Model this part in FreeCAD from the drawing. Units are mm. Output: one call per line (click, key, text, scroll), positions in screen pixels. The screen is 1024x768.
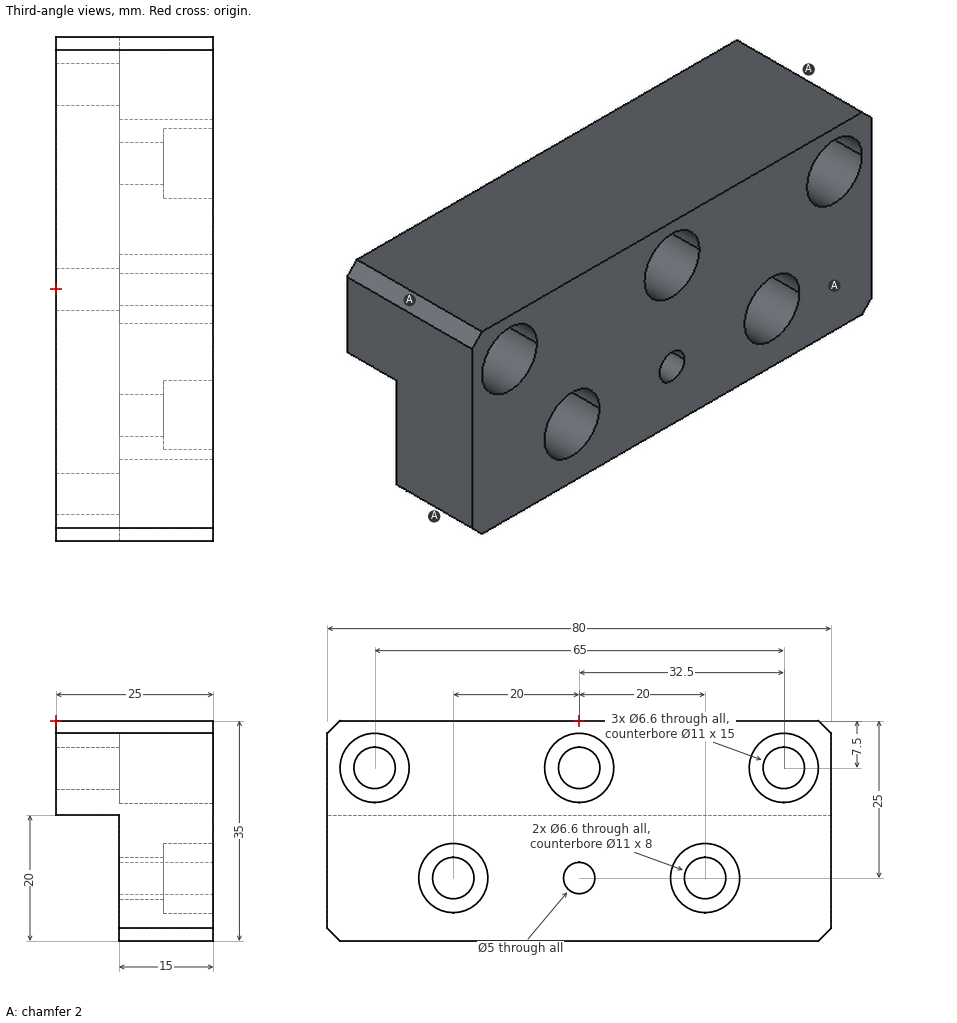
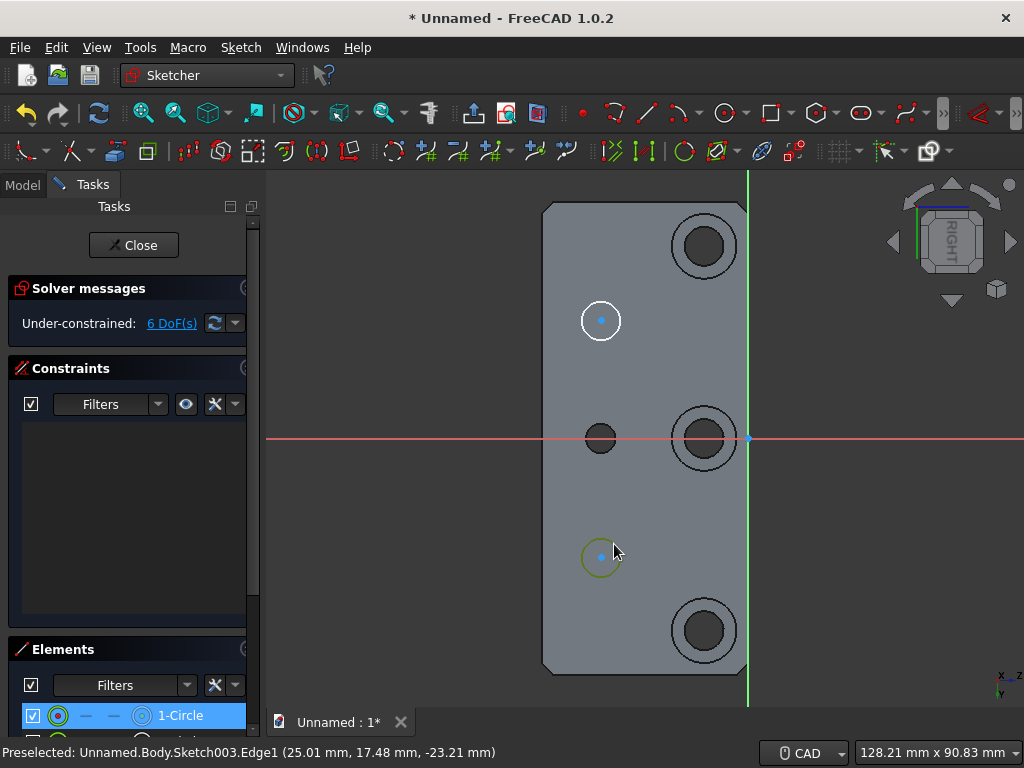
click(614, 307)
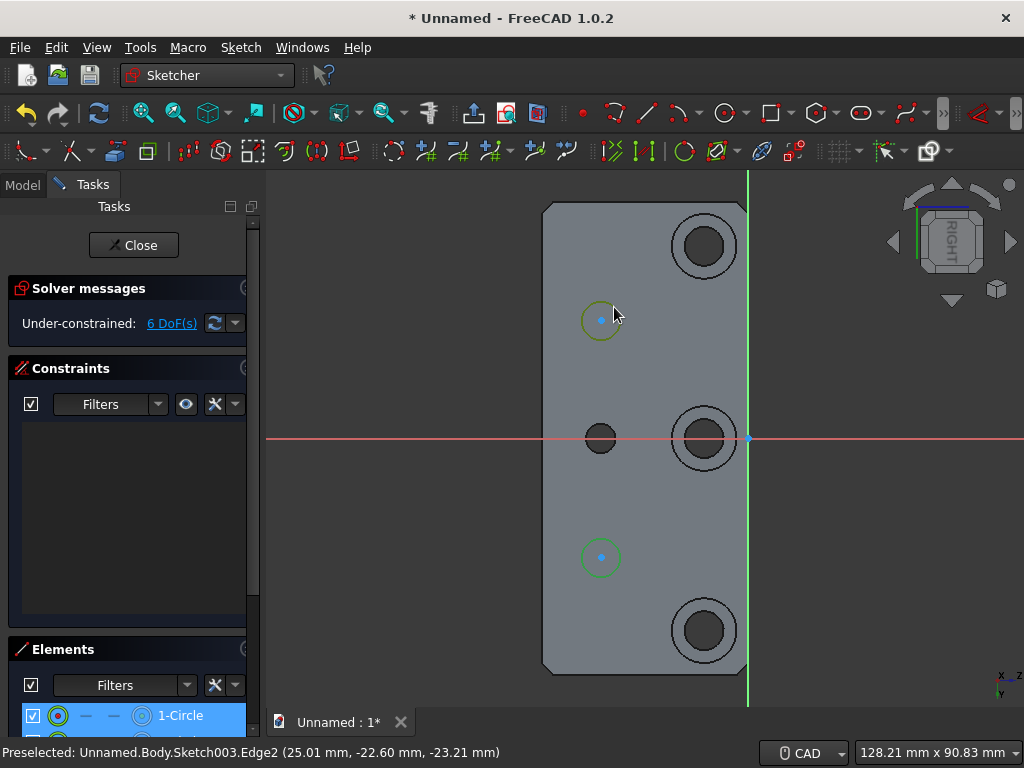
key(e)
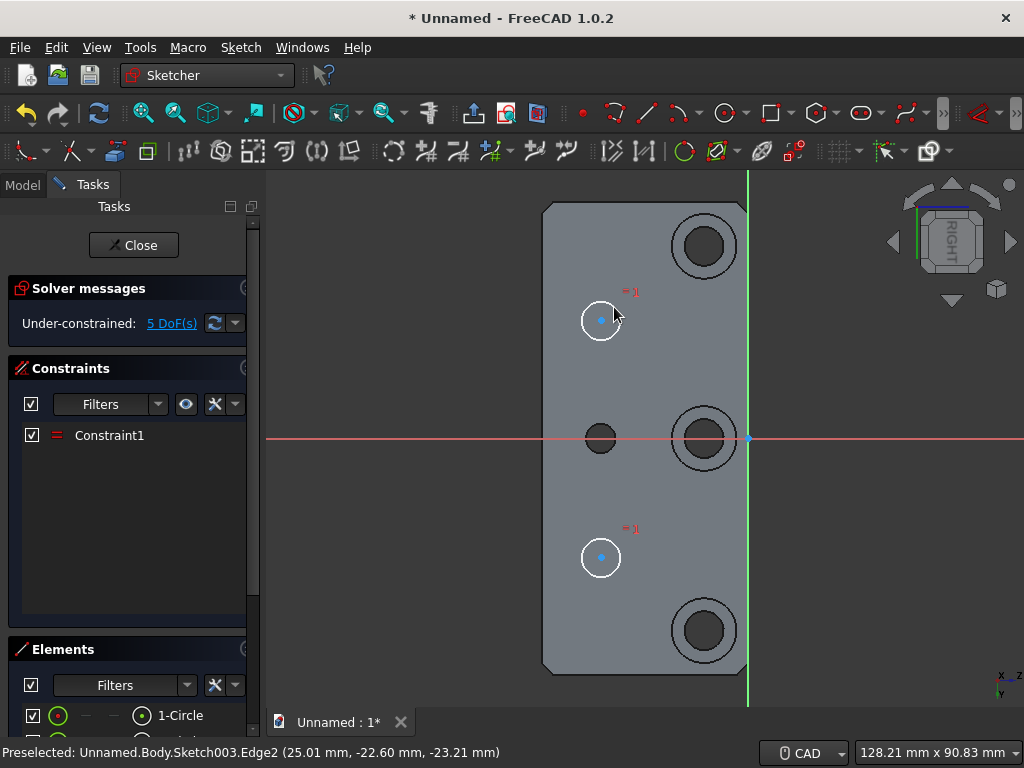
click(601, 558)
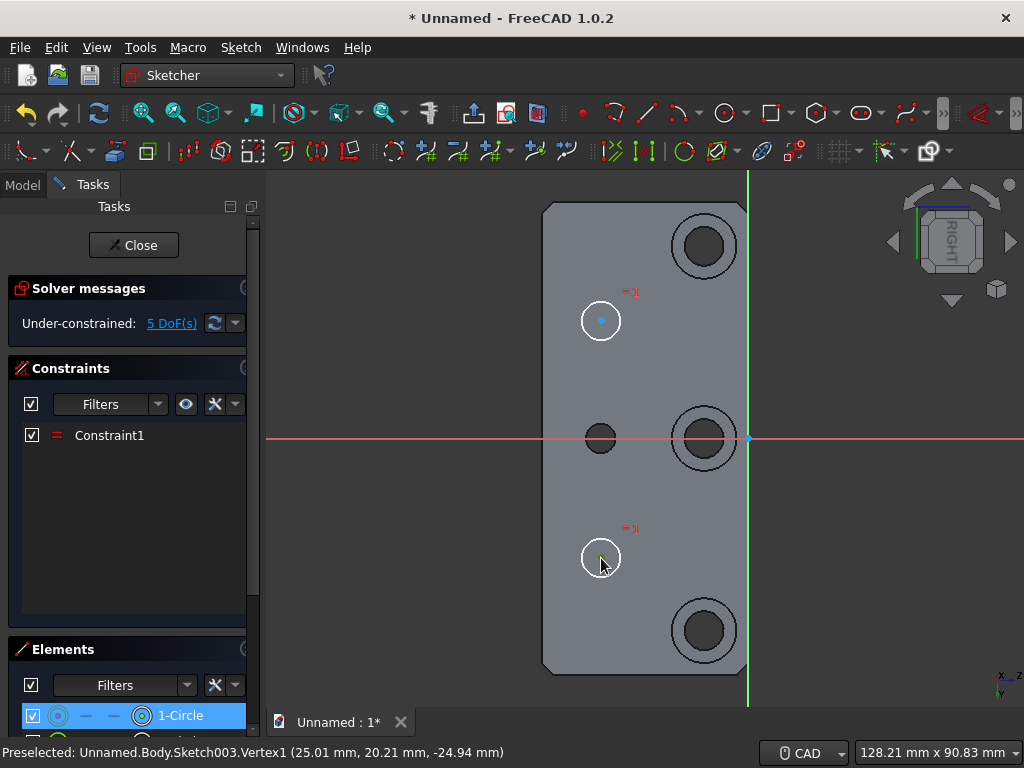
click(601, 321)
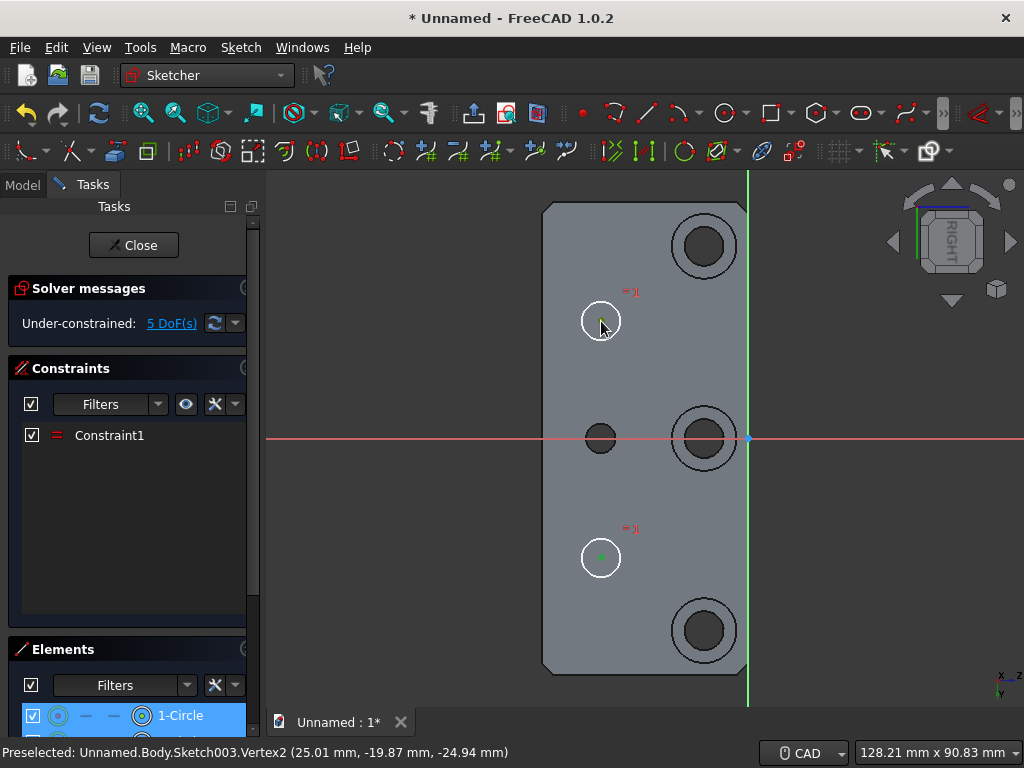
key(v)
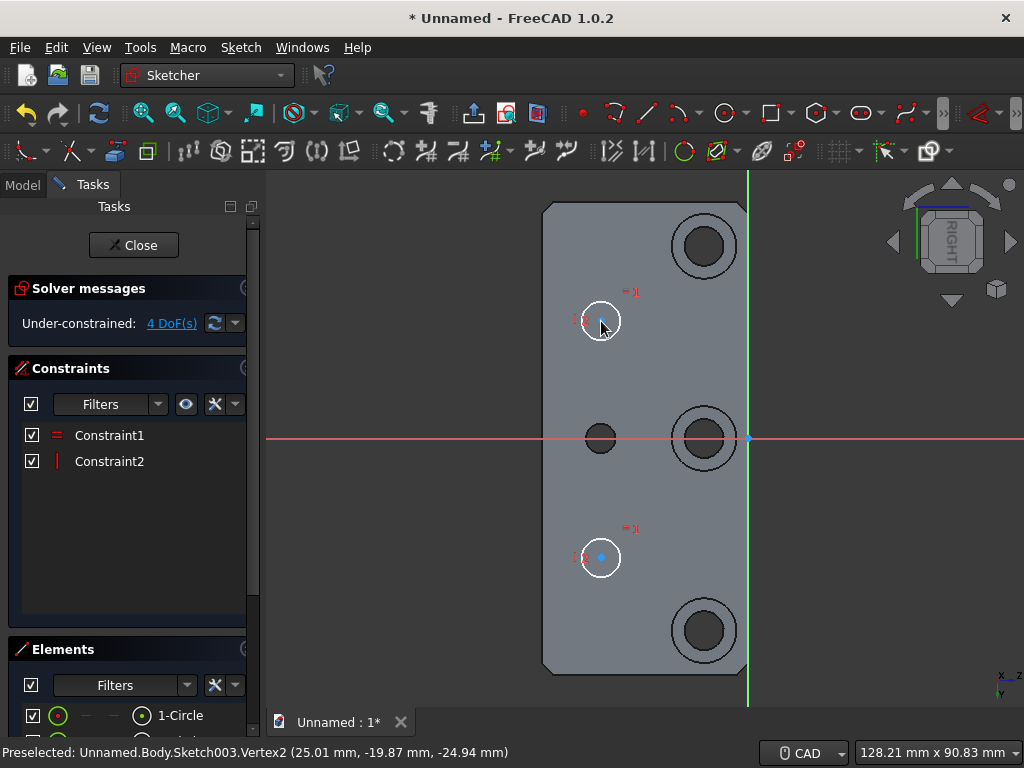
click(978, 114)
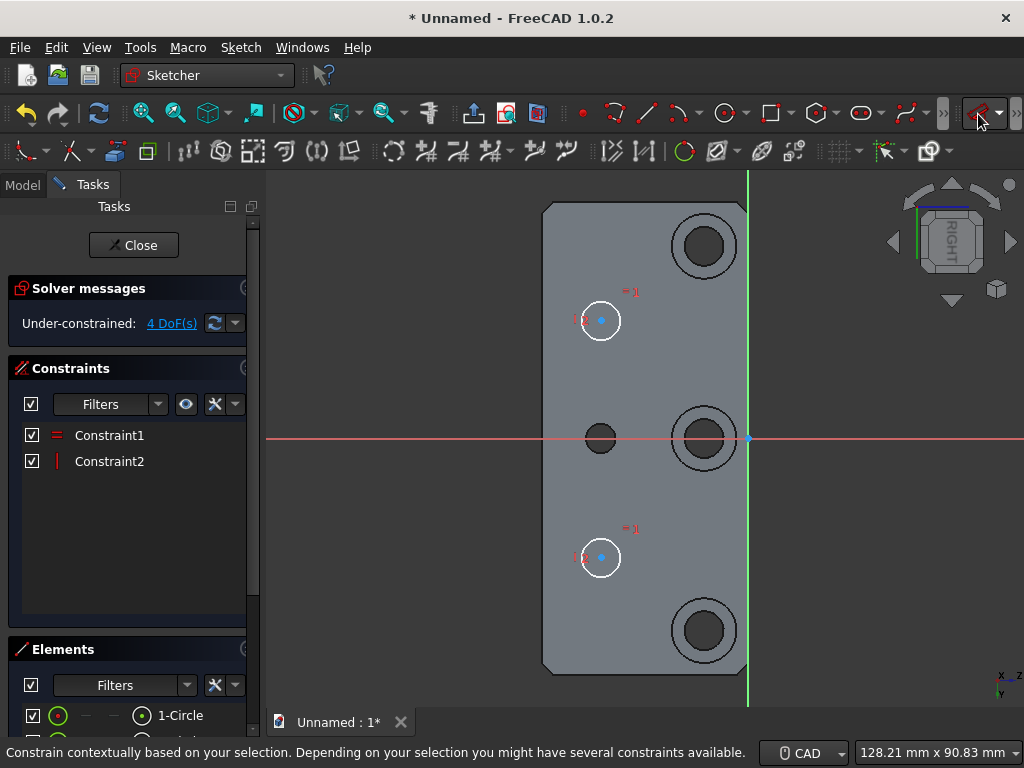
click(614, 544)
click(636, 521)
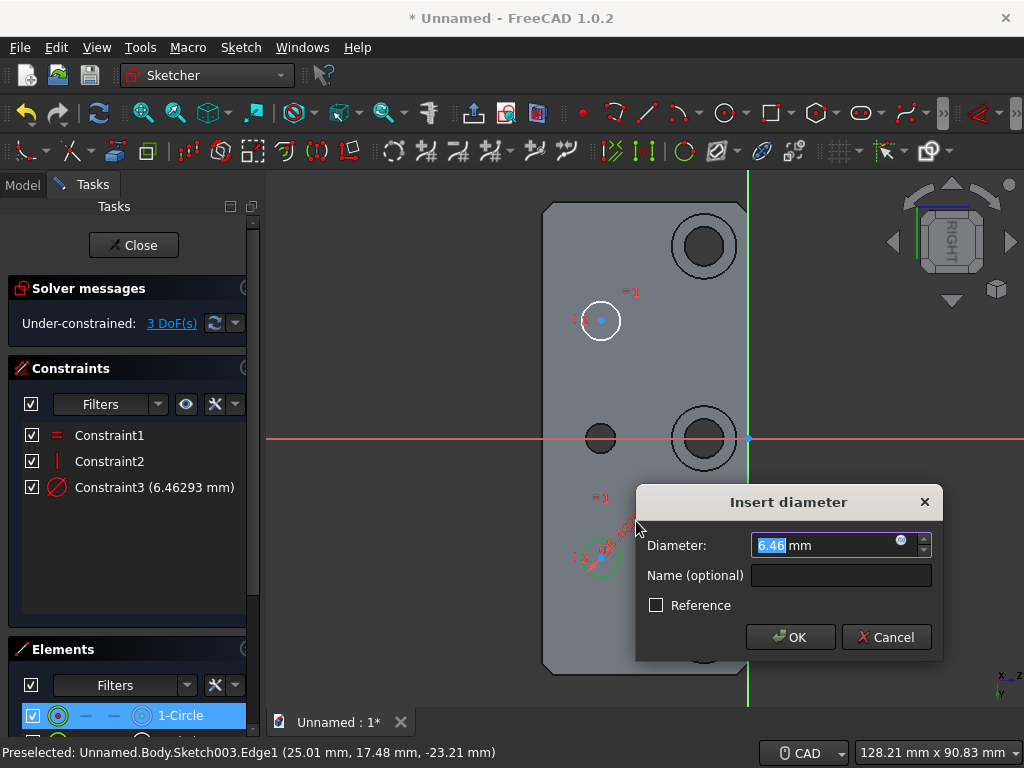
text(6.6)
key(Return)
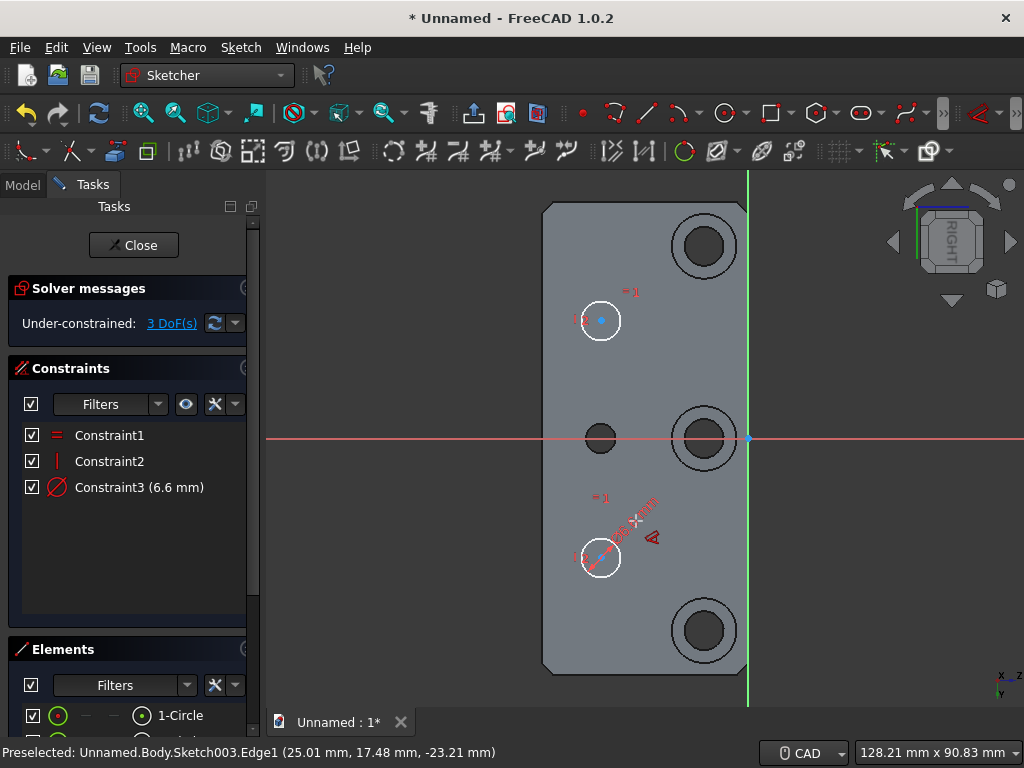
click(601, 558)
click(675, 592)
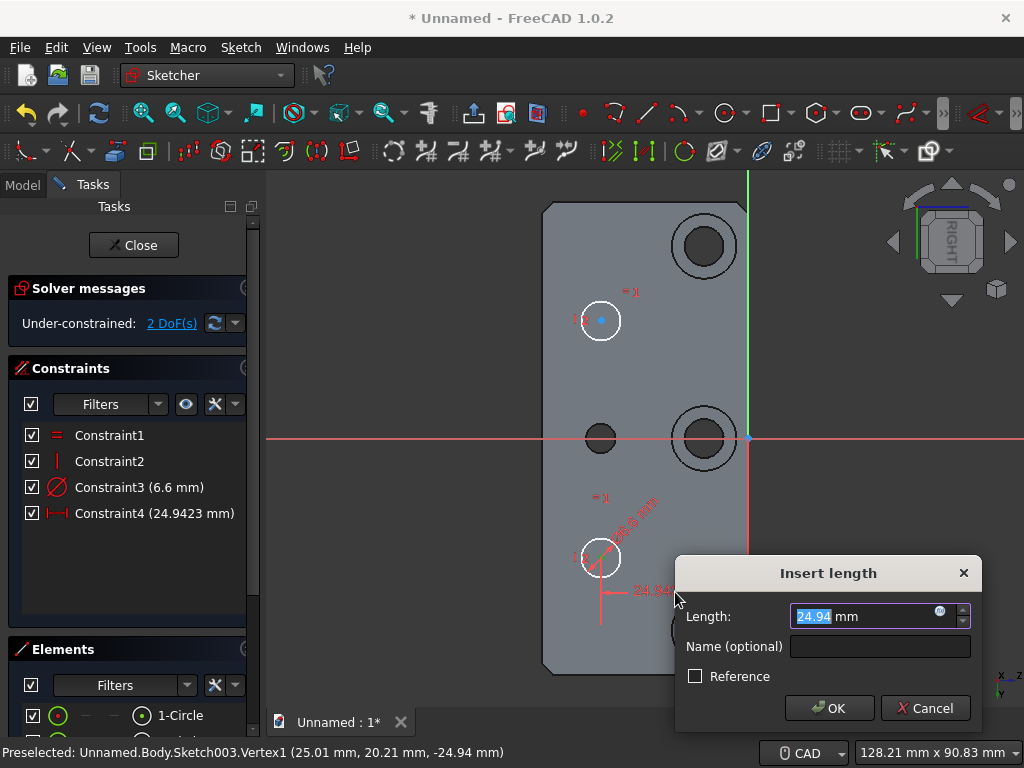
text(25)
key(Return)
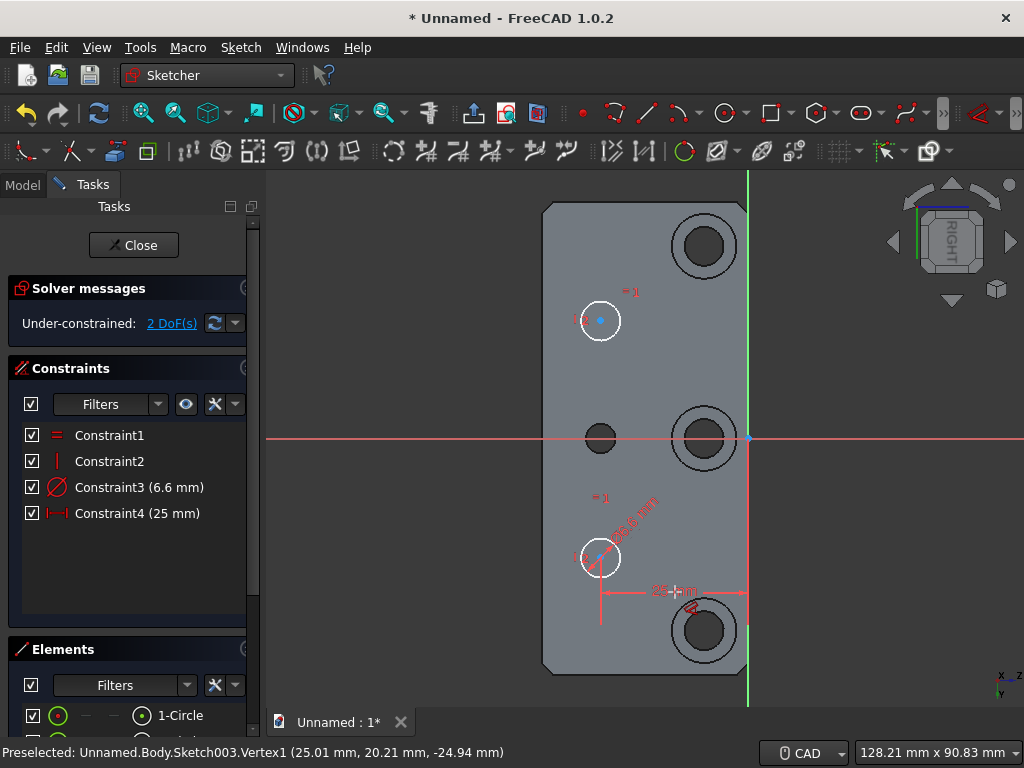
click(601, 558)
click(782, 498)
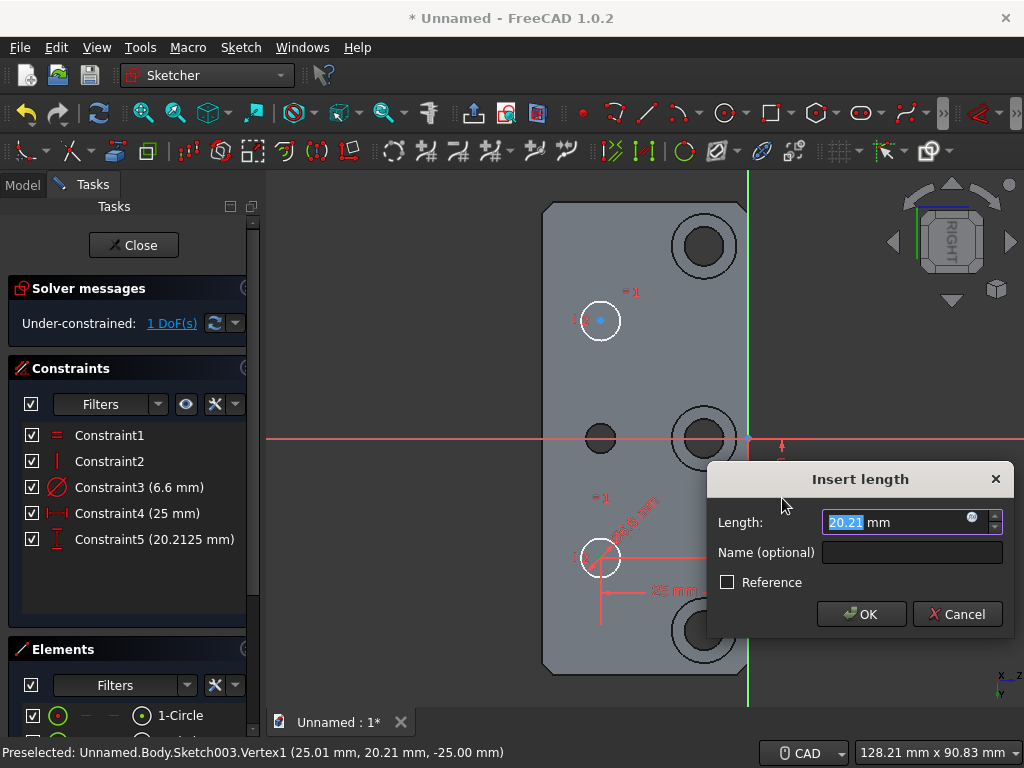
text(20)
key(Return)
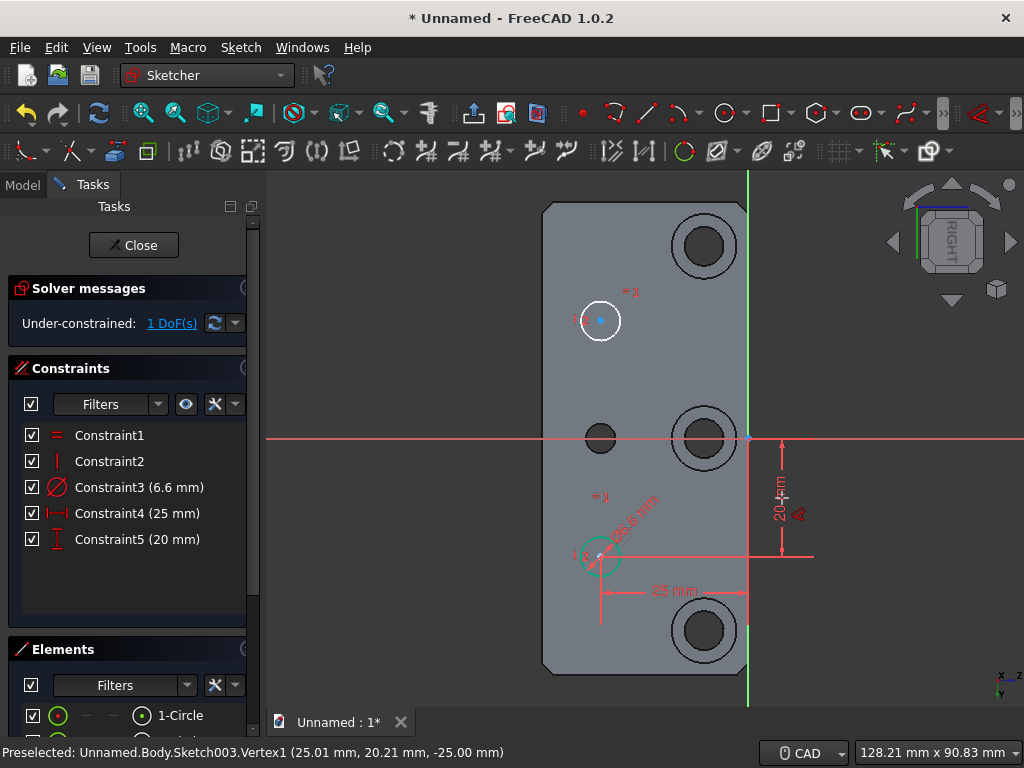
click(601, 321)
click(782, 380)